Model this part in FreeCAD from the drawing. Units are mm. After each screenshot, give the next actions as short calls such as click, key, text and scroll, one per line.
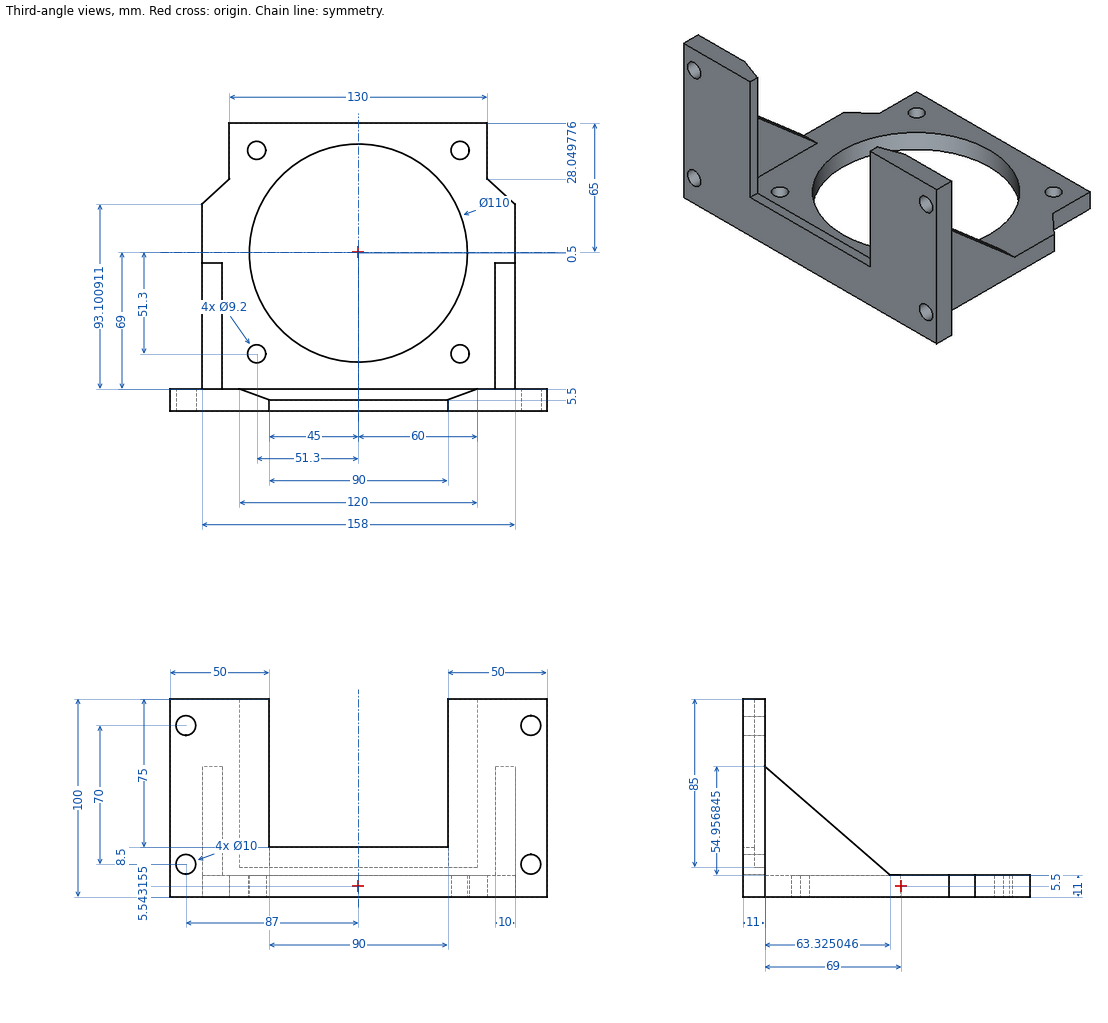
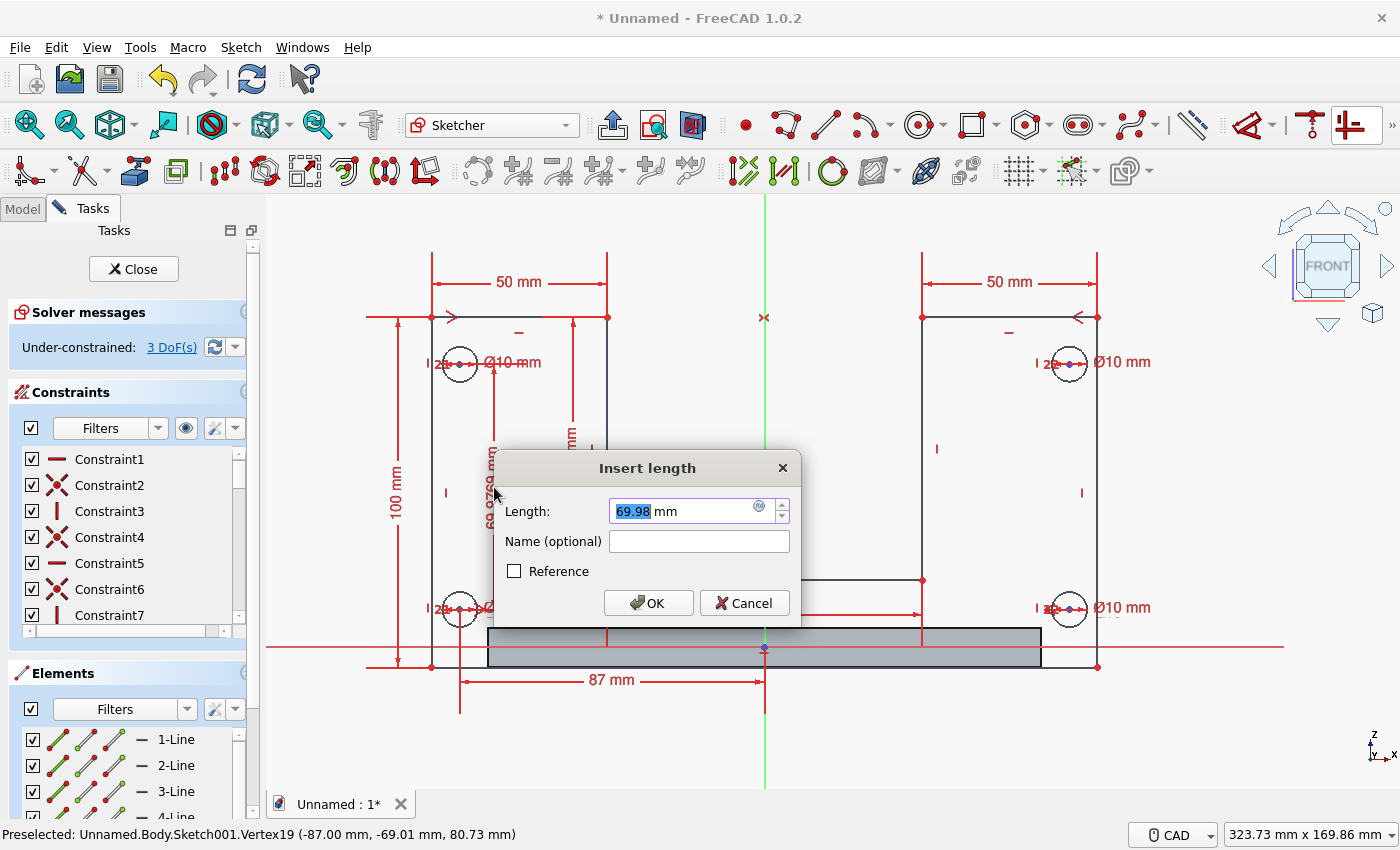
text(70)
key(Return)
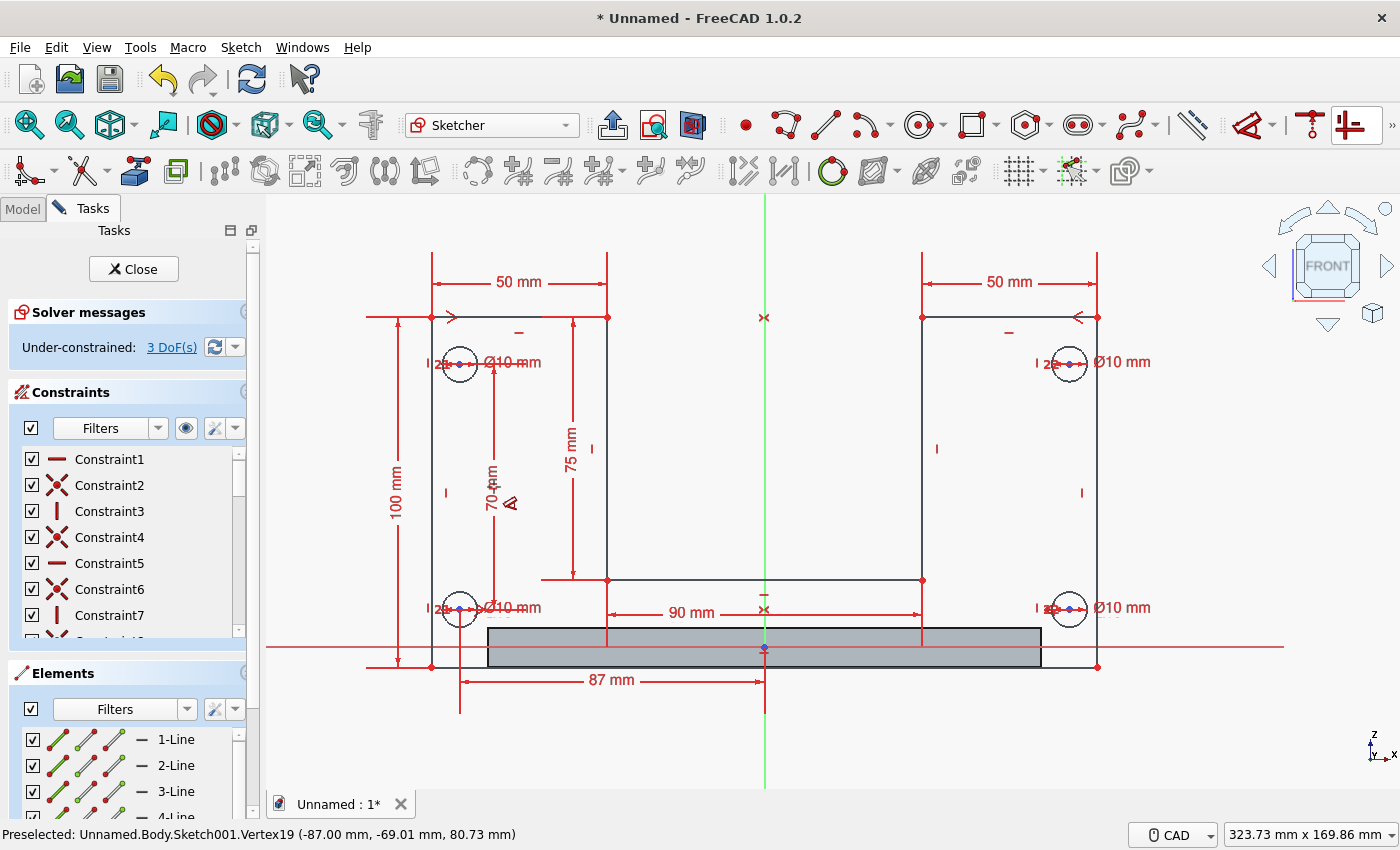
click(1069, 610)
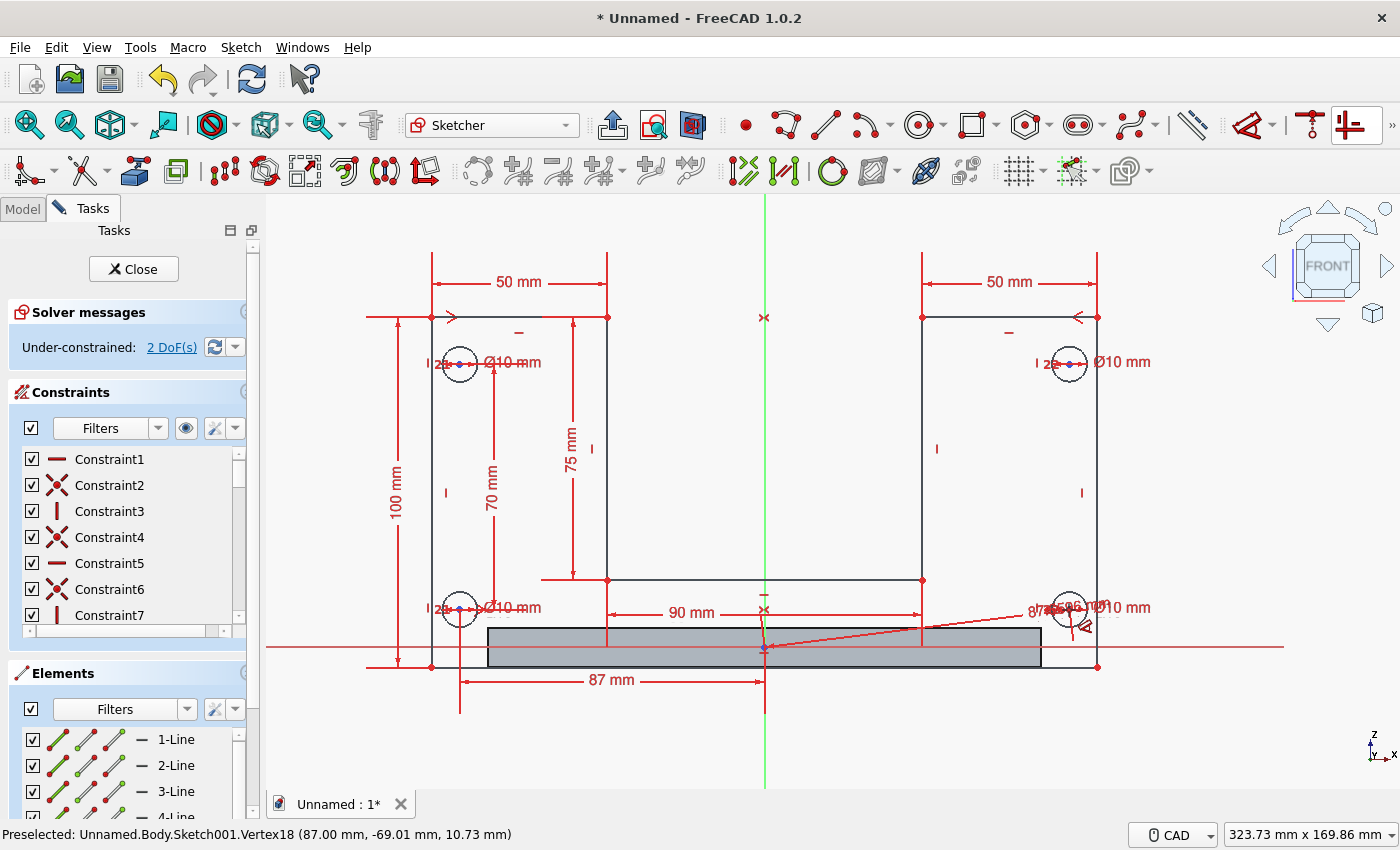
click(1069, 364)
click(1035, 487)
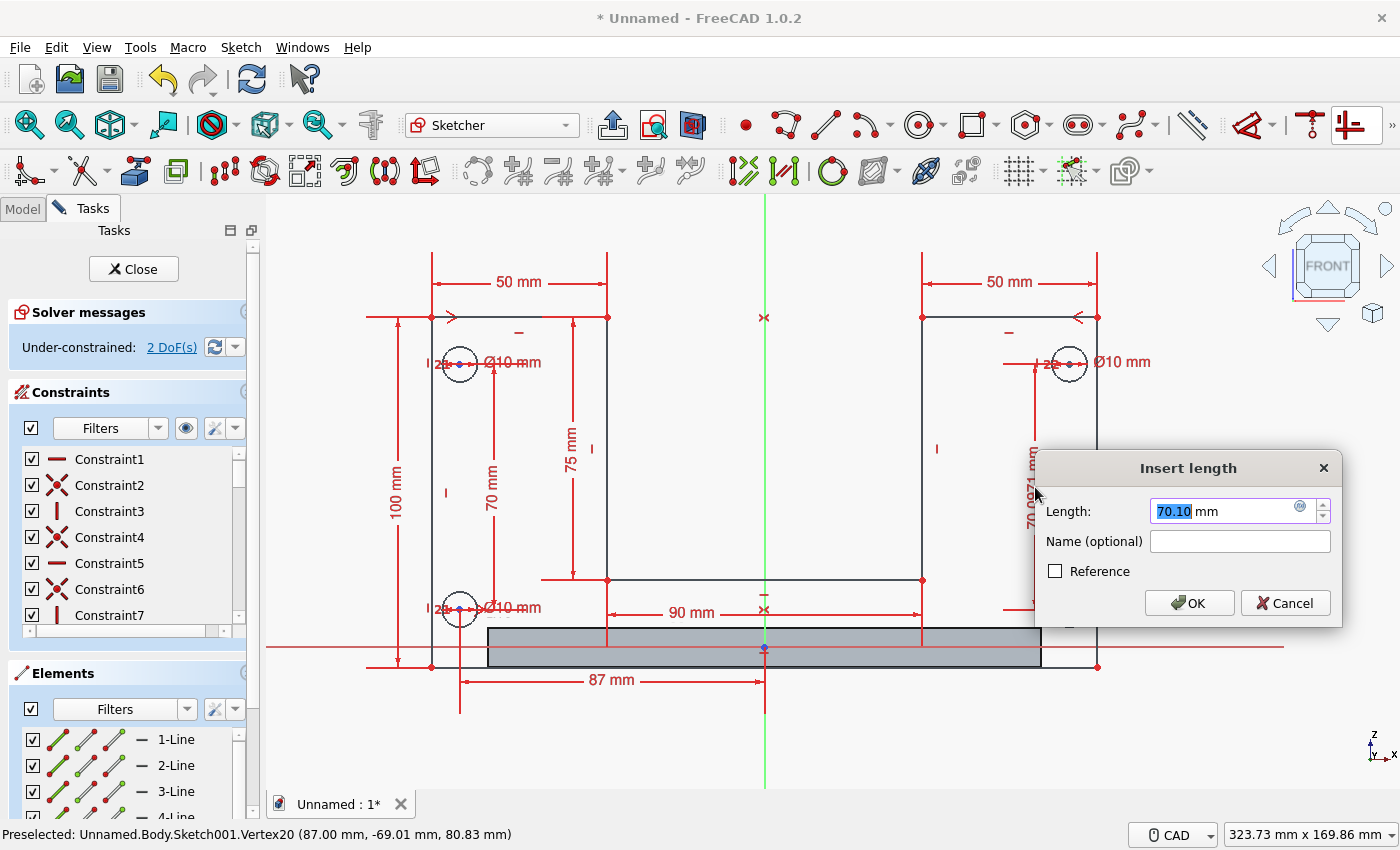
text(70)
key(Return)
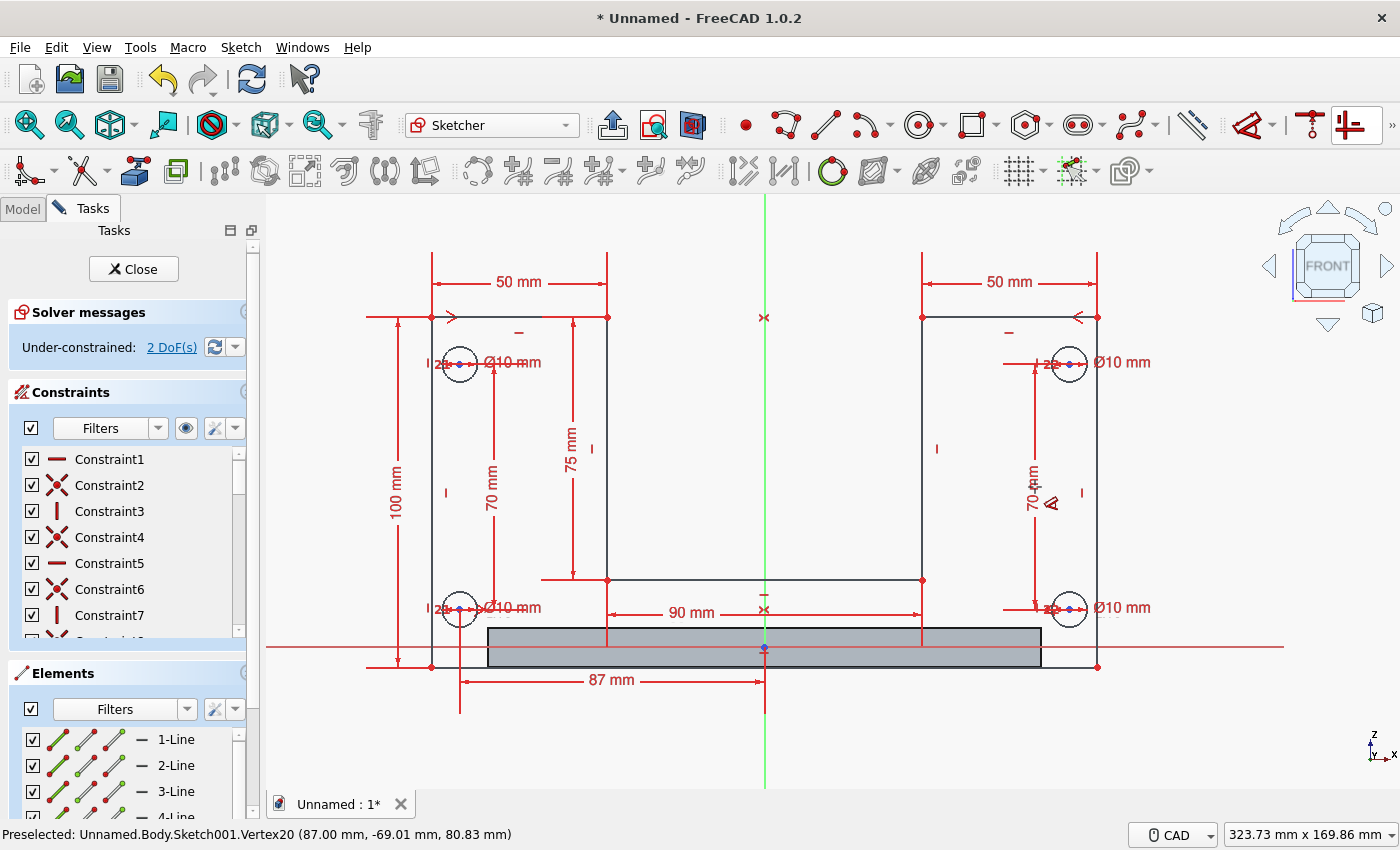
scroll(607, 580, up, 2)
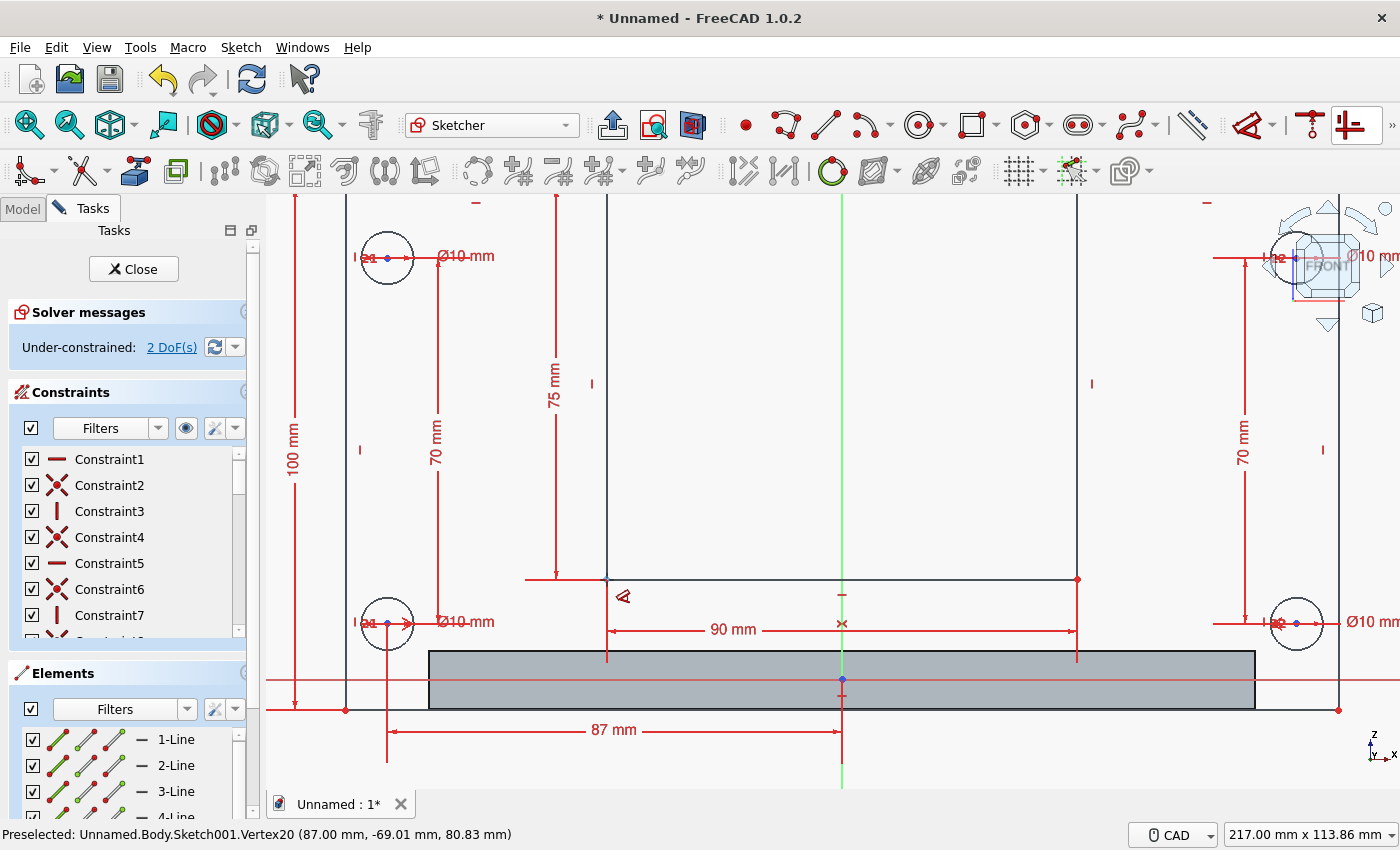
click(607, 580)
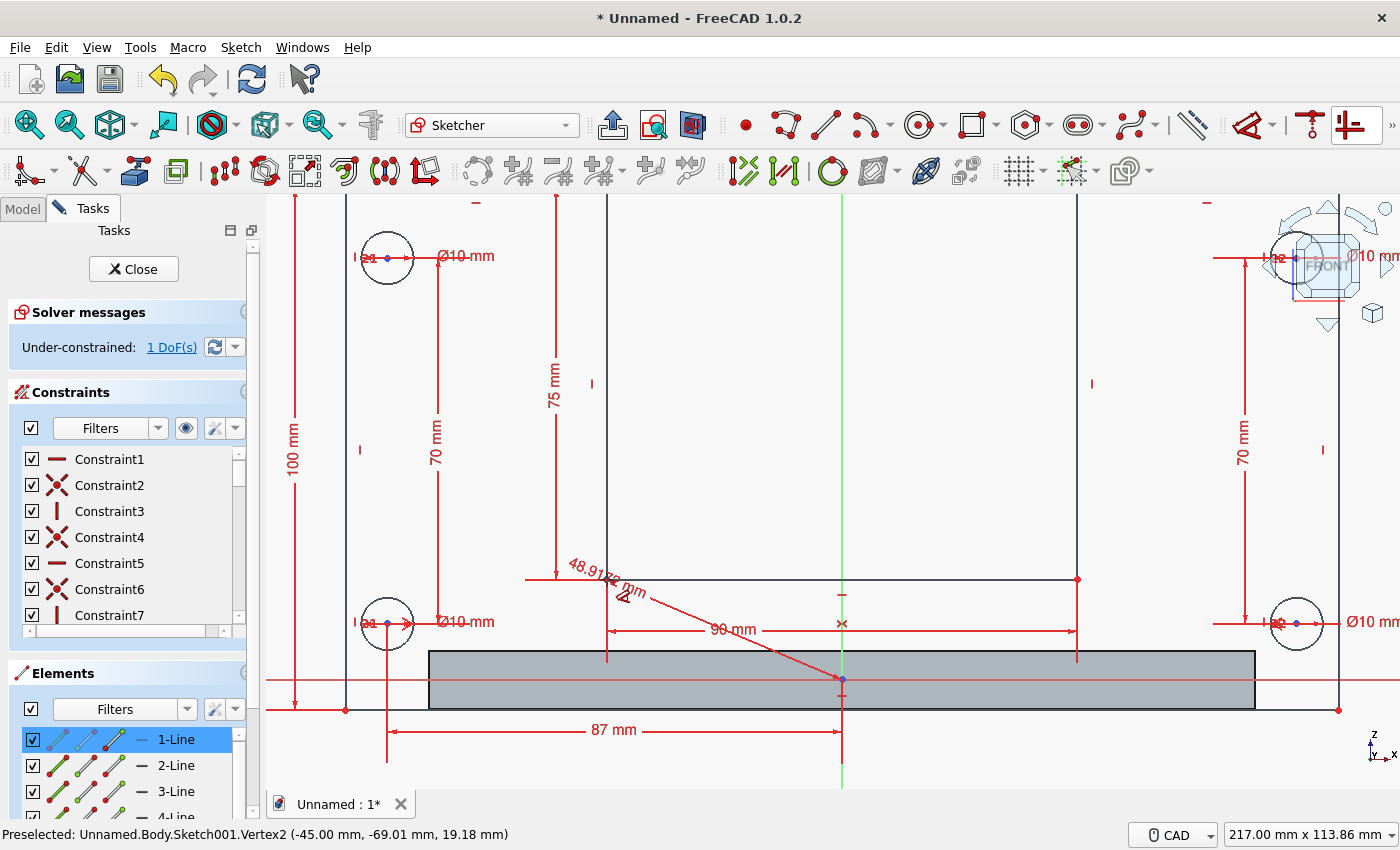
click(387, 624)
click(641, 602)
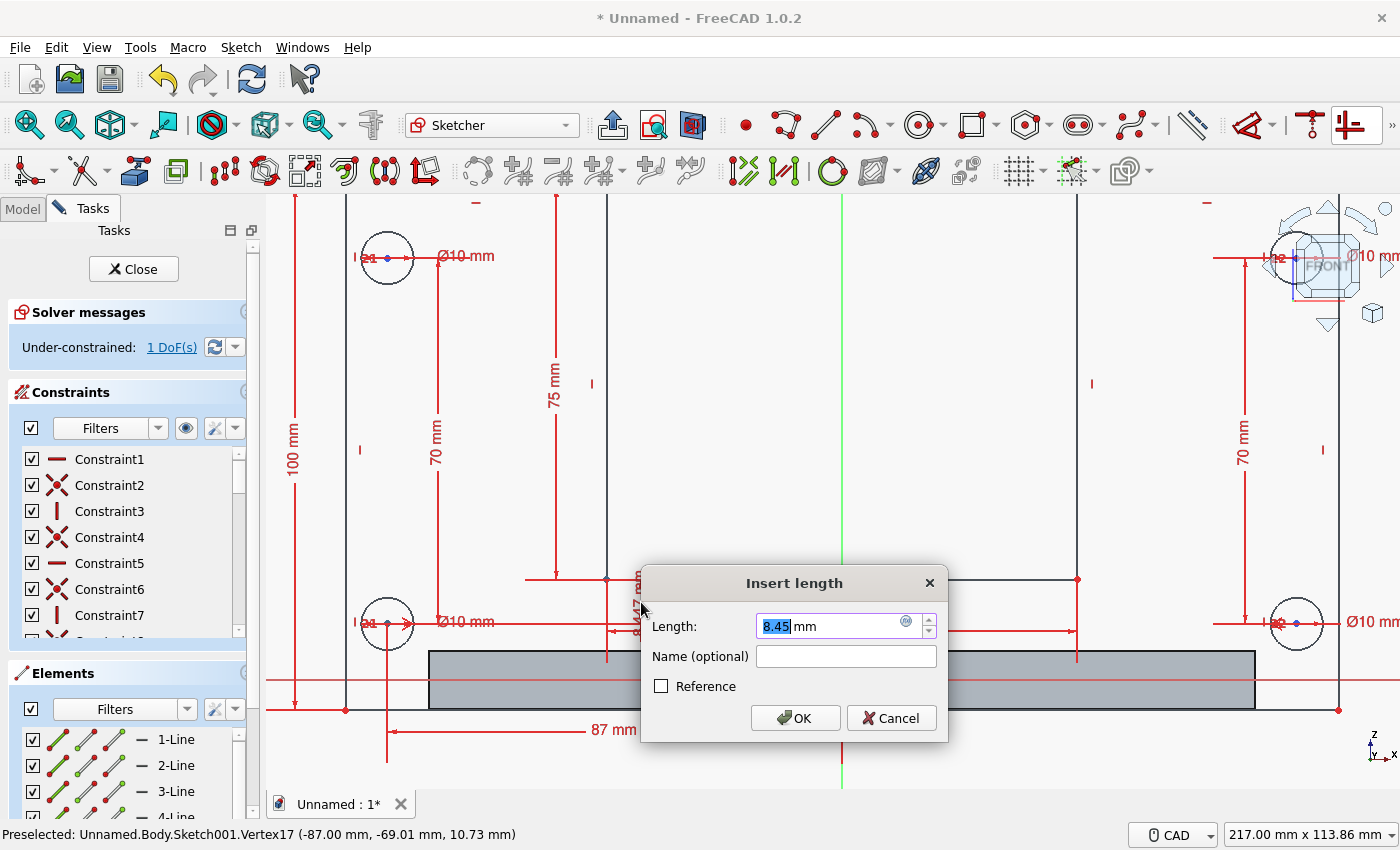
text(8.5)
key(Return)